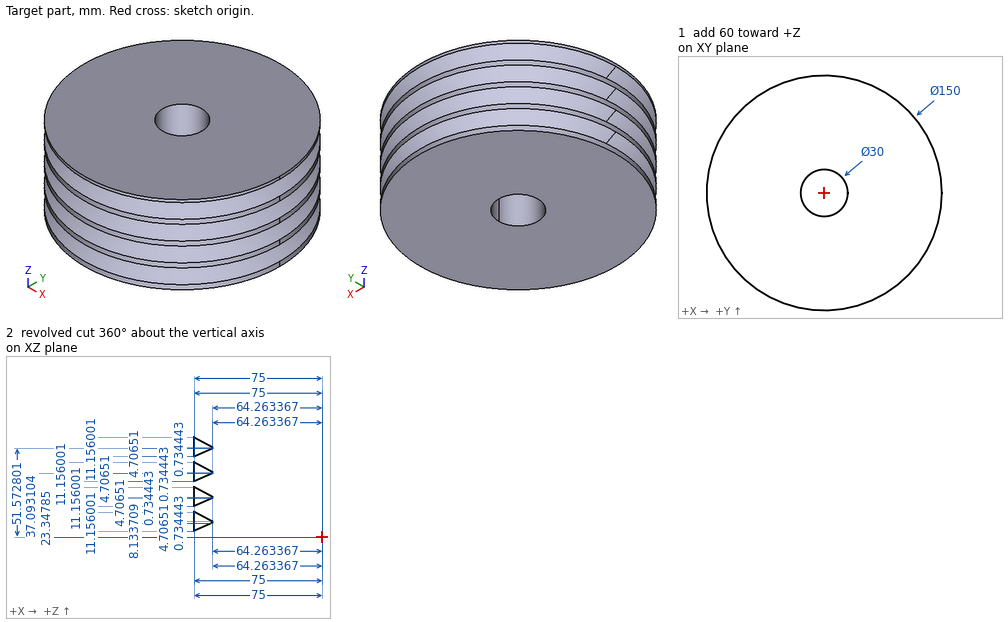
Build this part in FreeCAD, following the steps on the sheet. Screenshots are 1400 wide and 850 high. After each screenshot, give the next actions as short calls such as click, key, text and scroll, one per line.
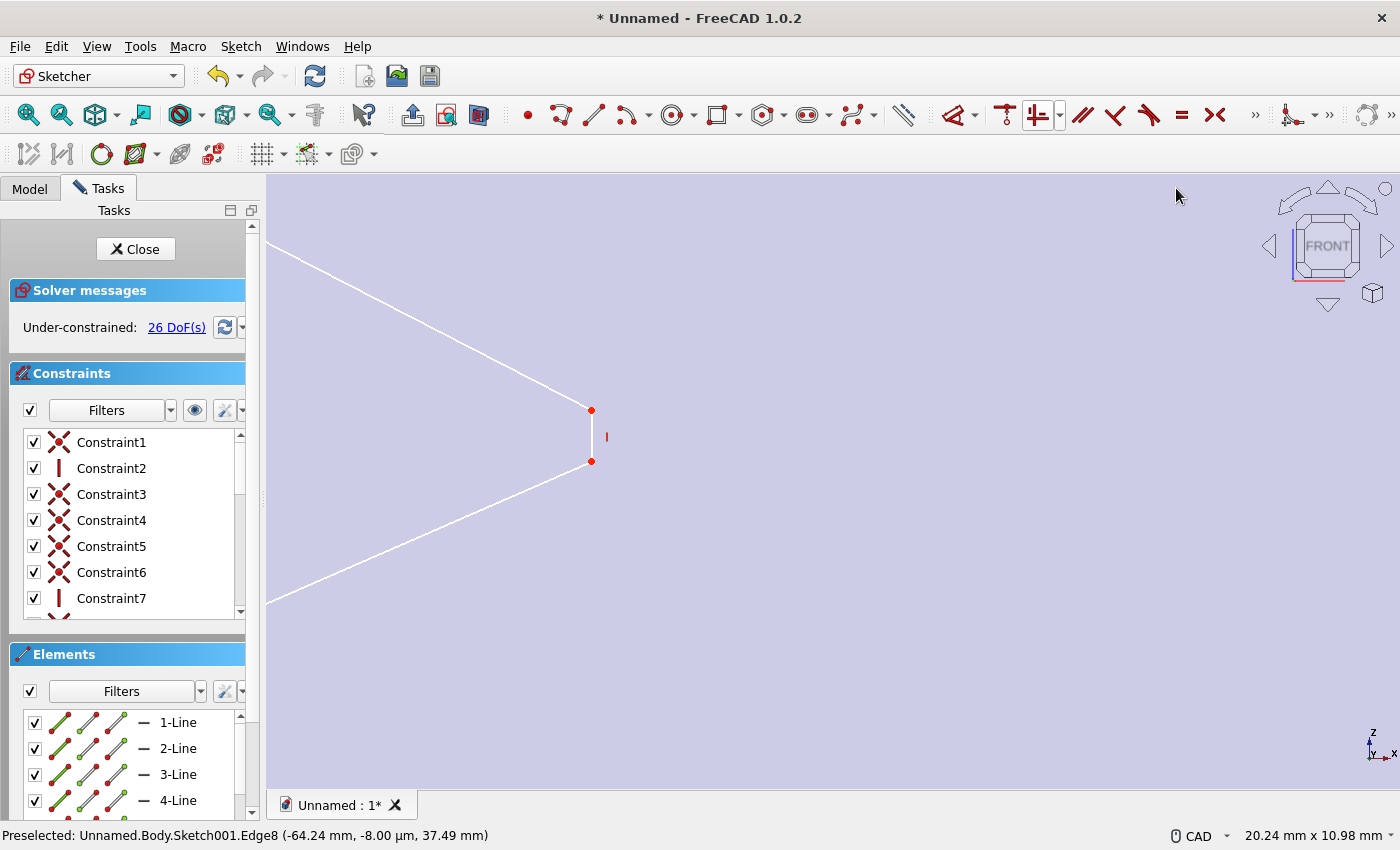
scroll(599, 429, down, 11)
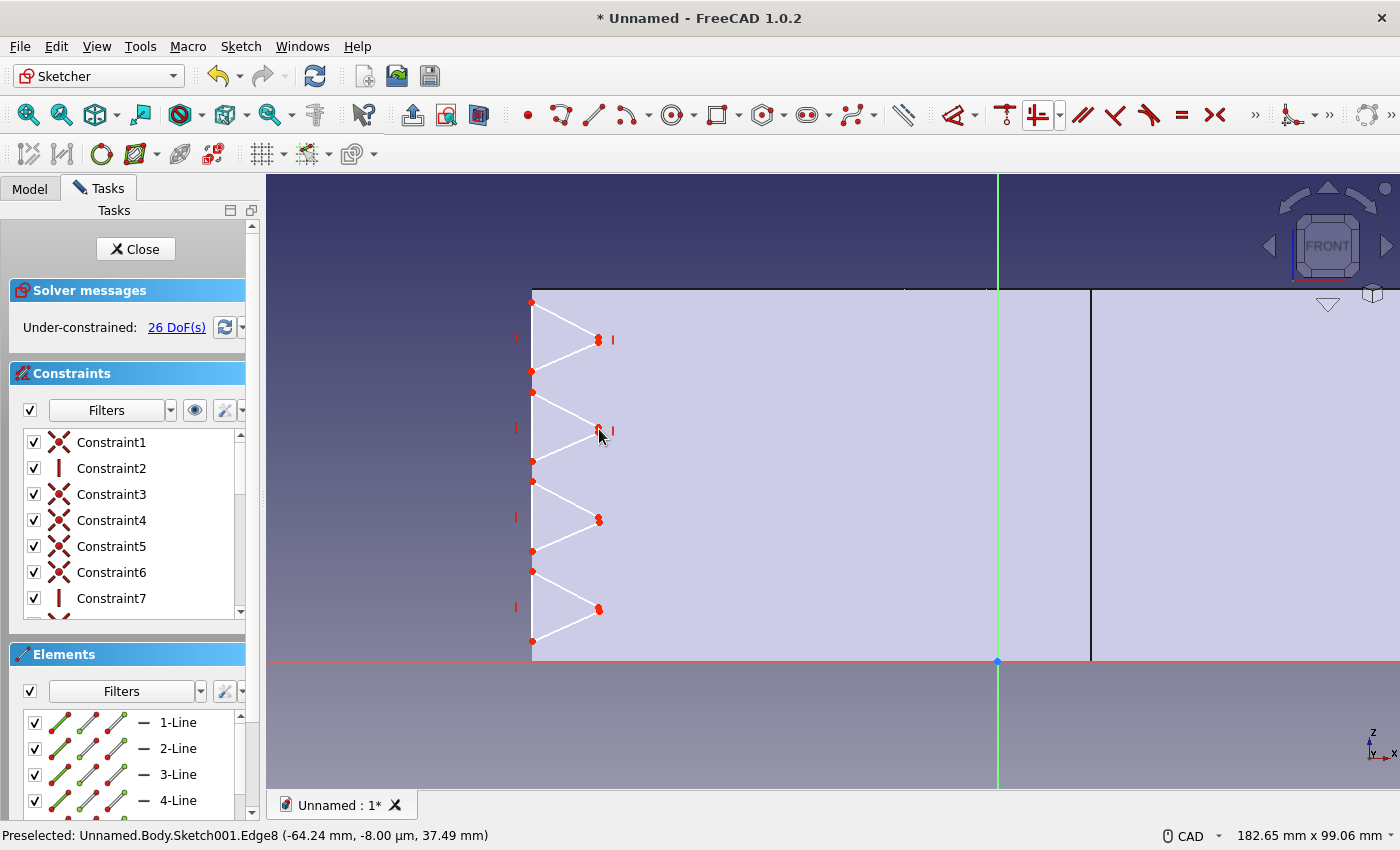
scroll(599, 519, up, 11)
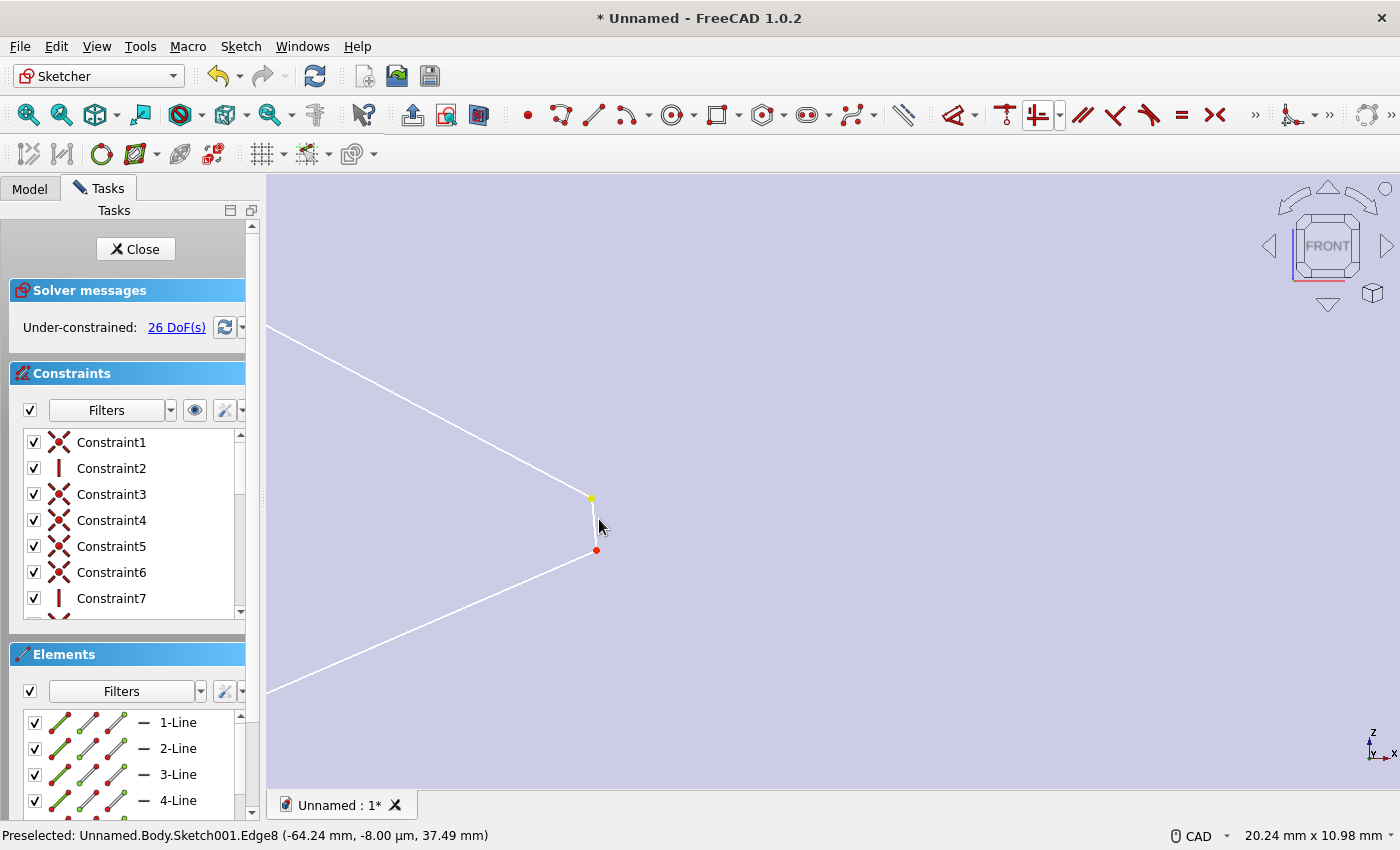
click(593, 514)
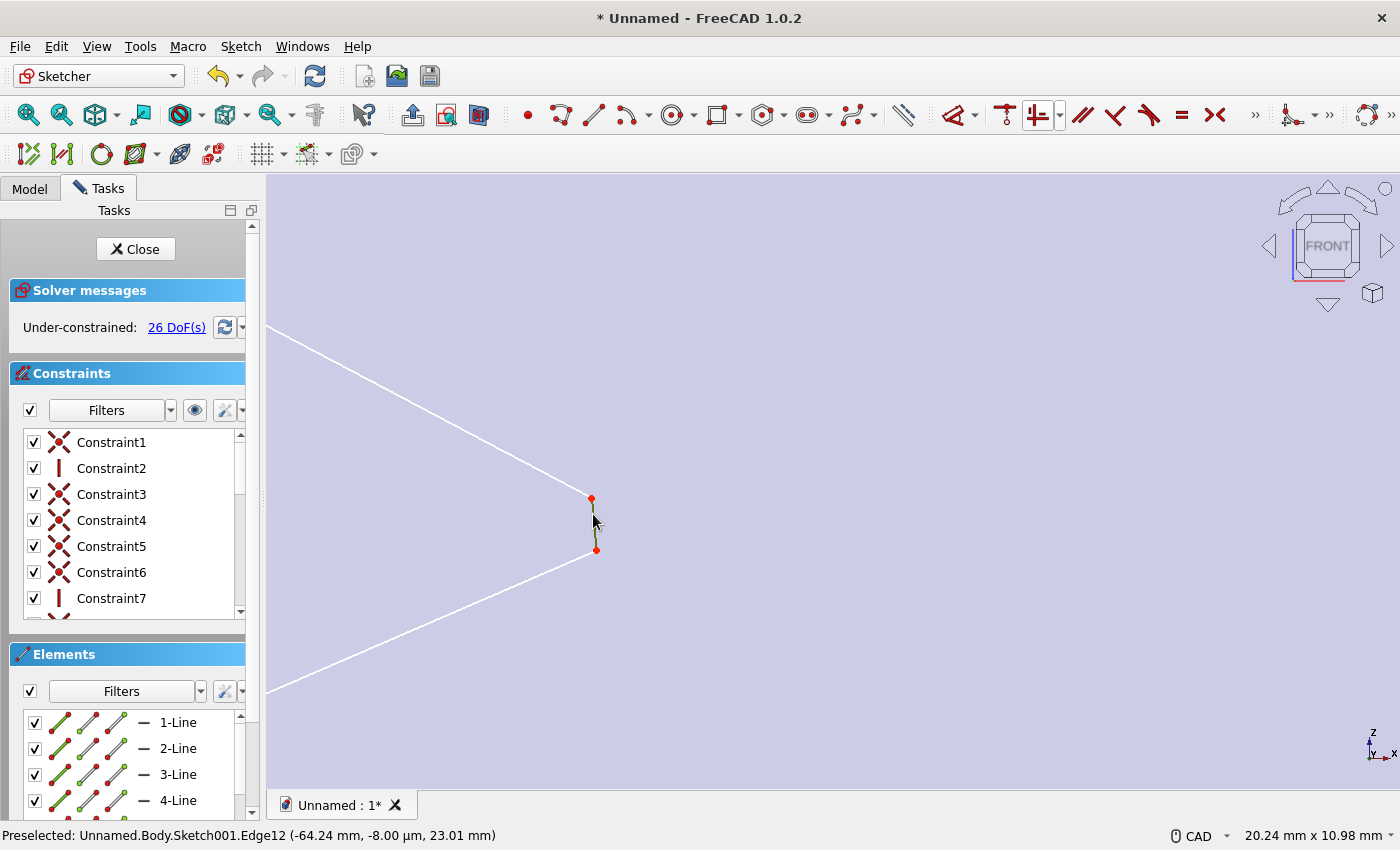
click(1060, 116)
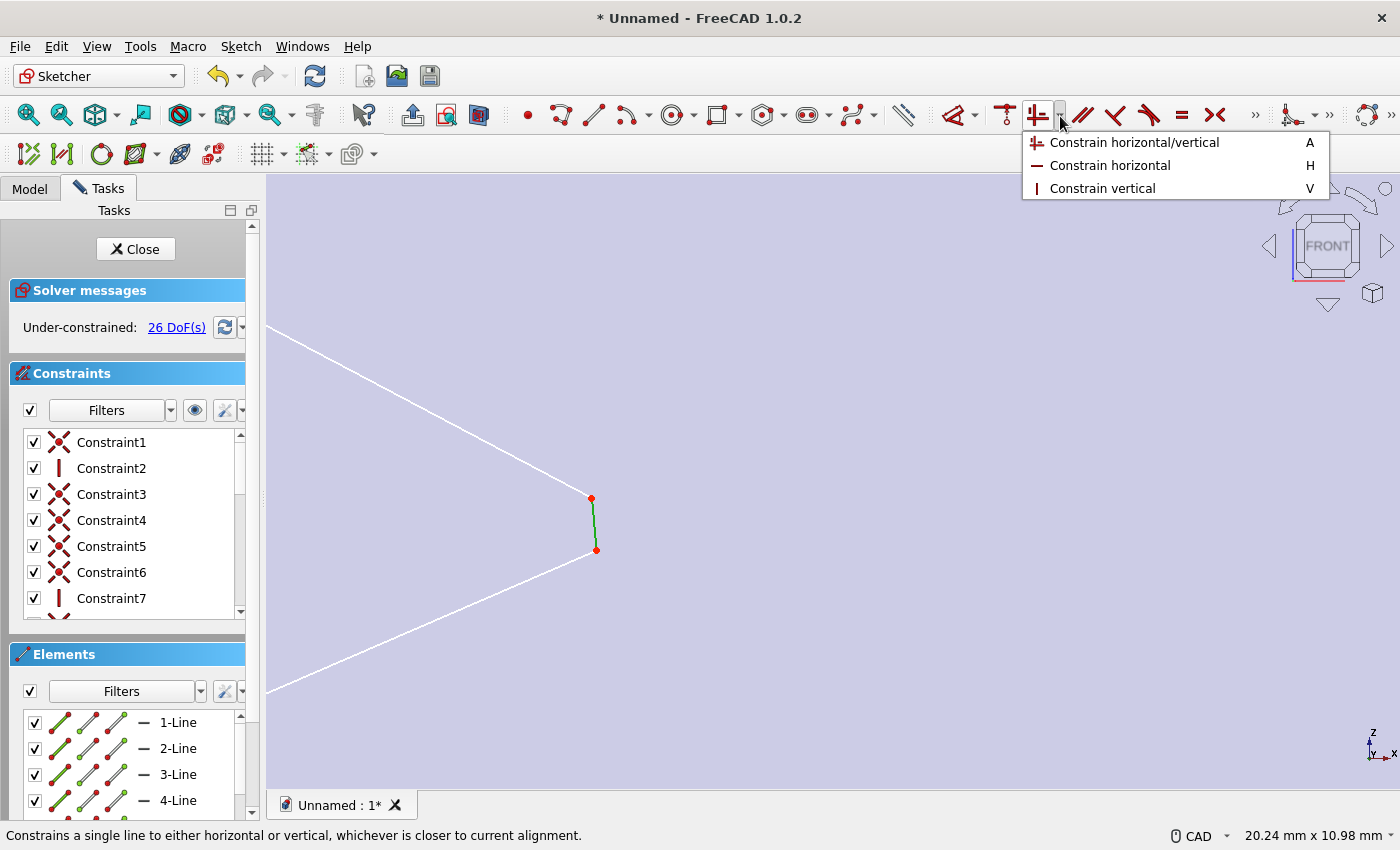
click(1176, 188)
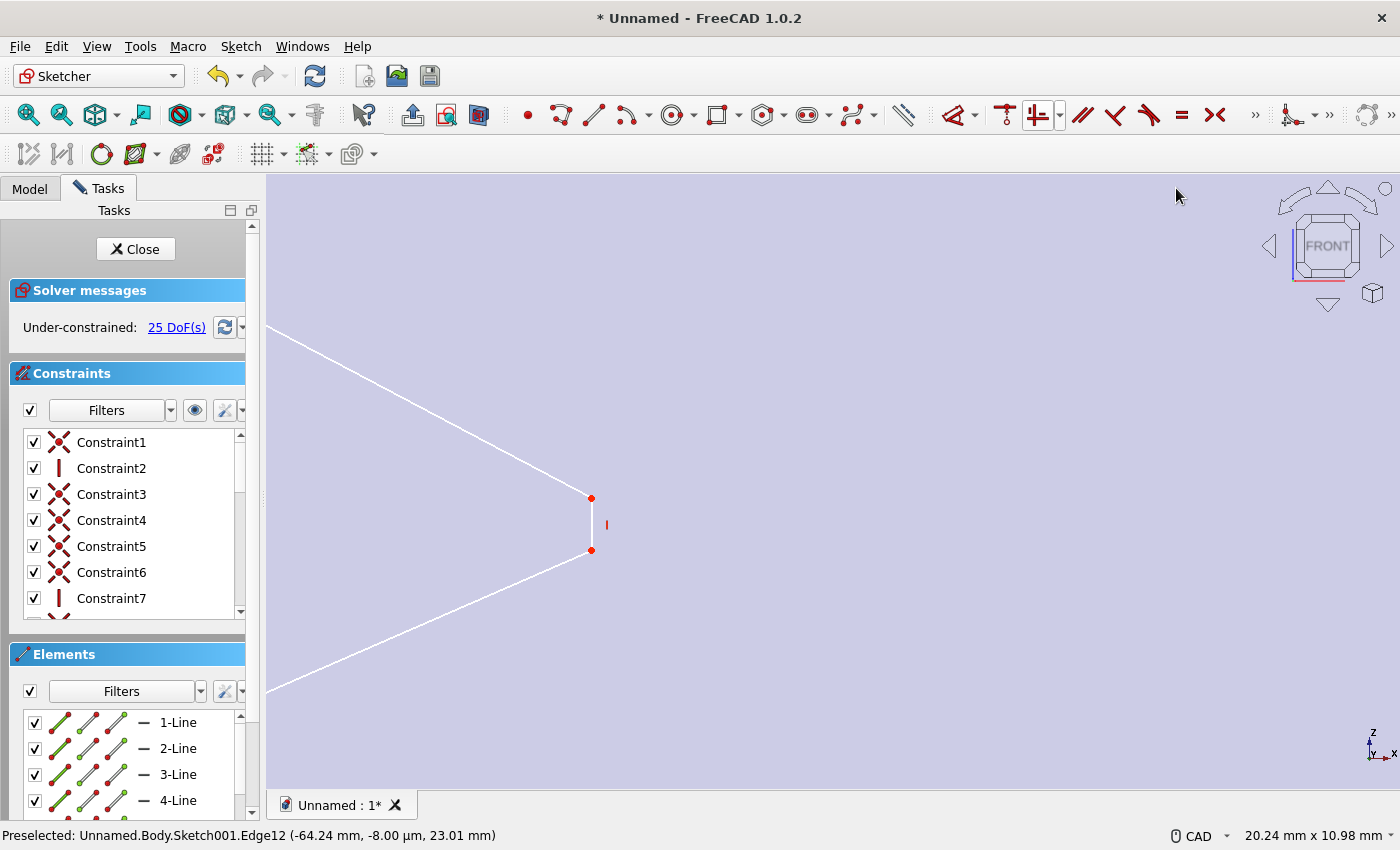
scroll(599, 519, down, 11)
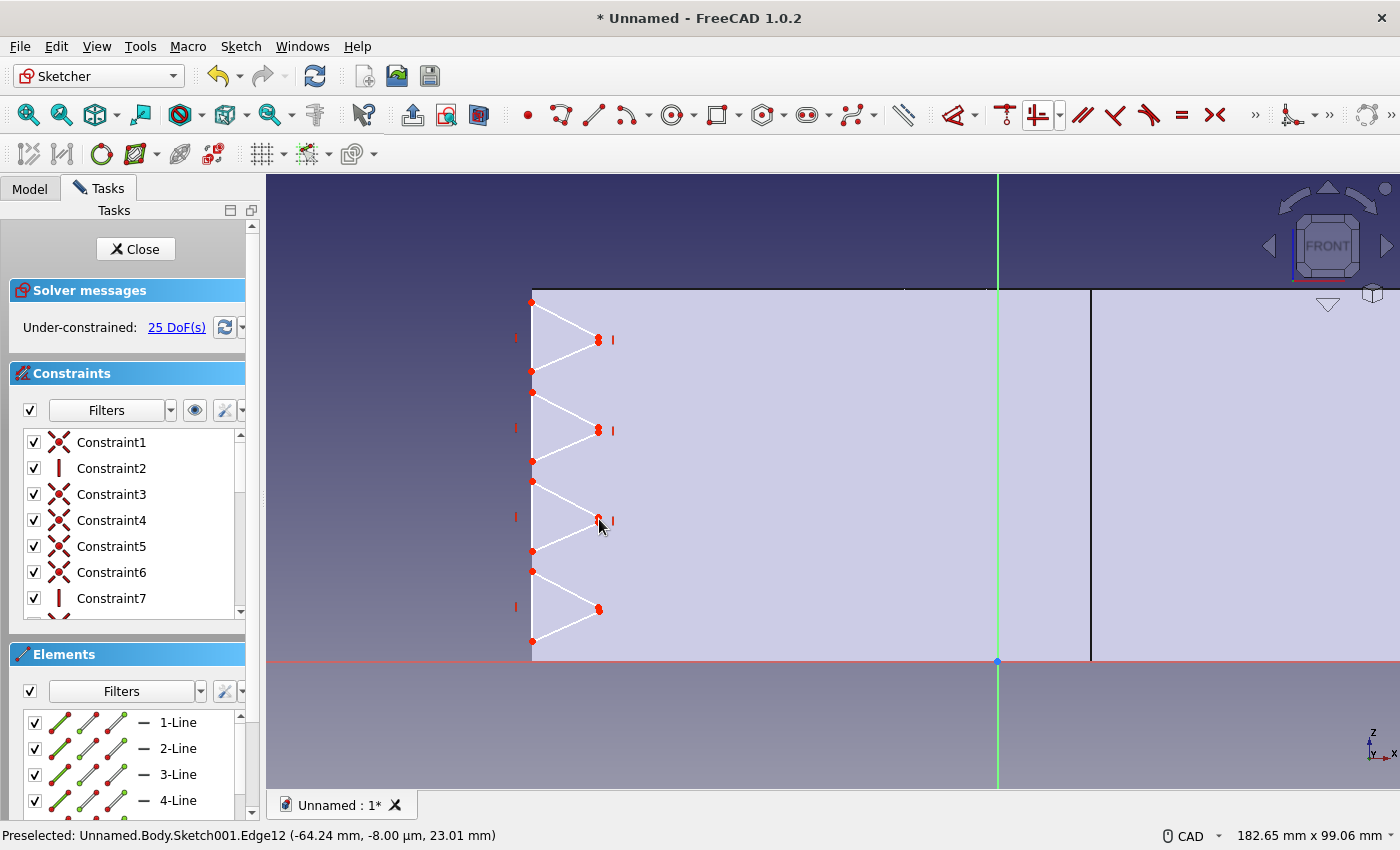
scroll(599, 609, up, 12)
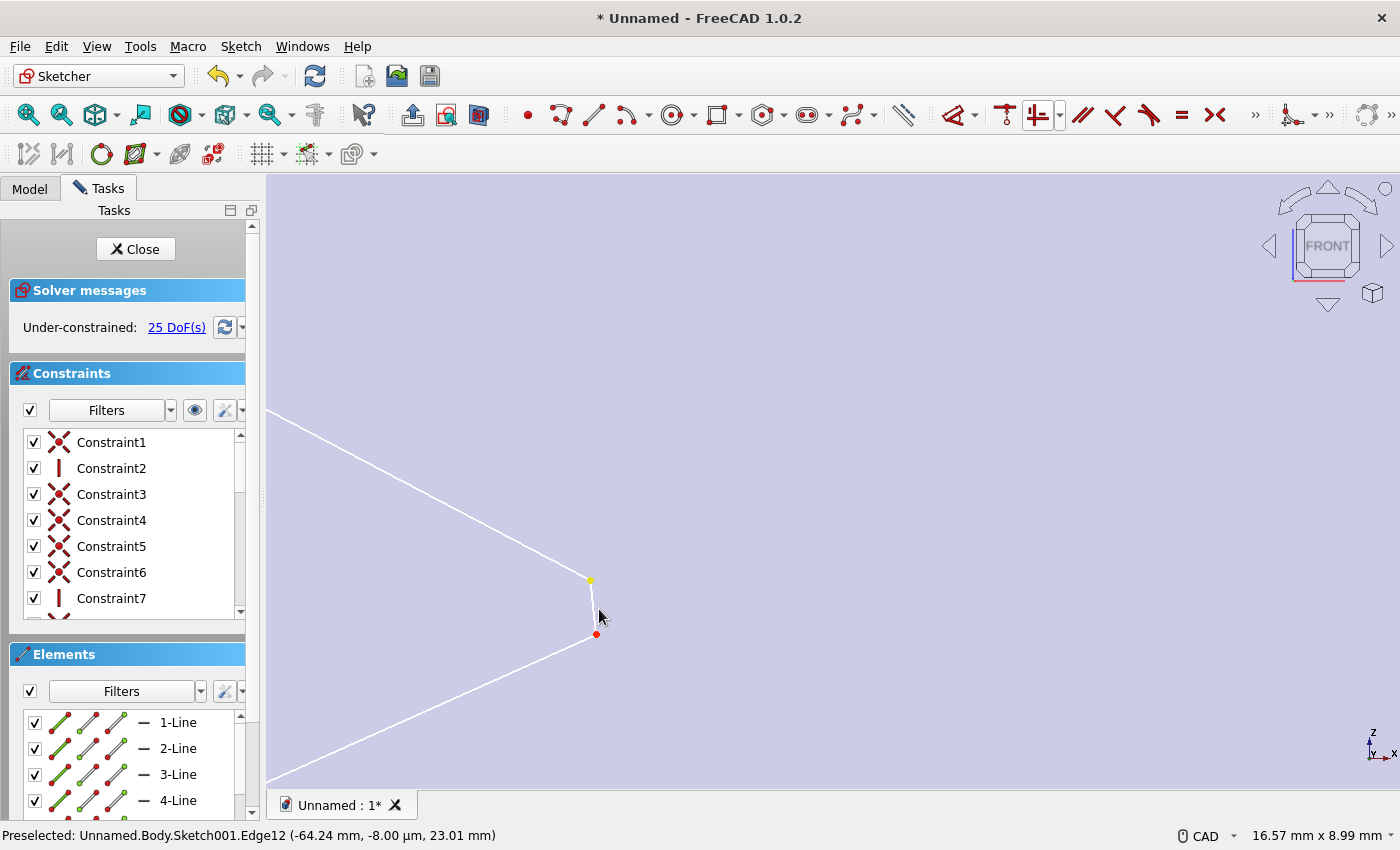
click(592, 597)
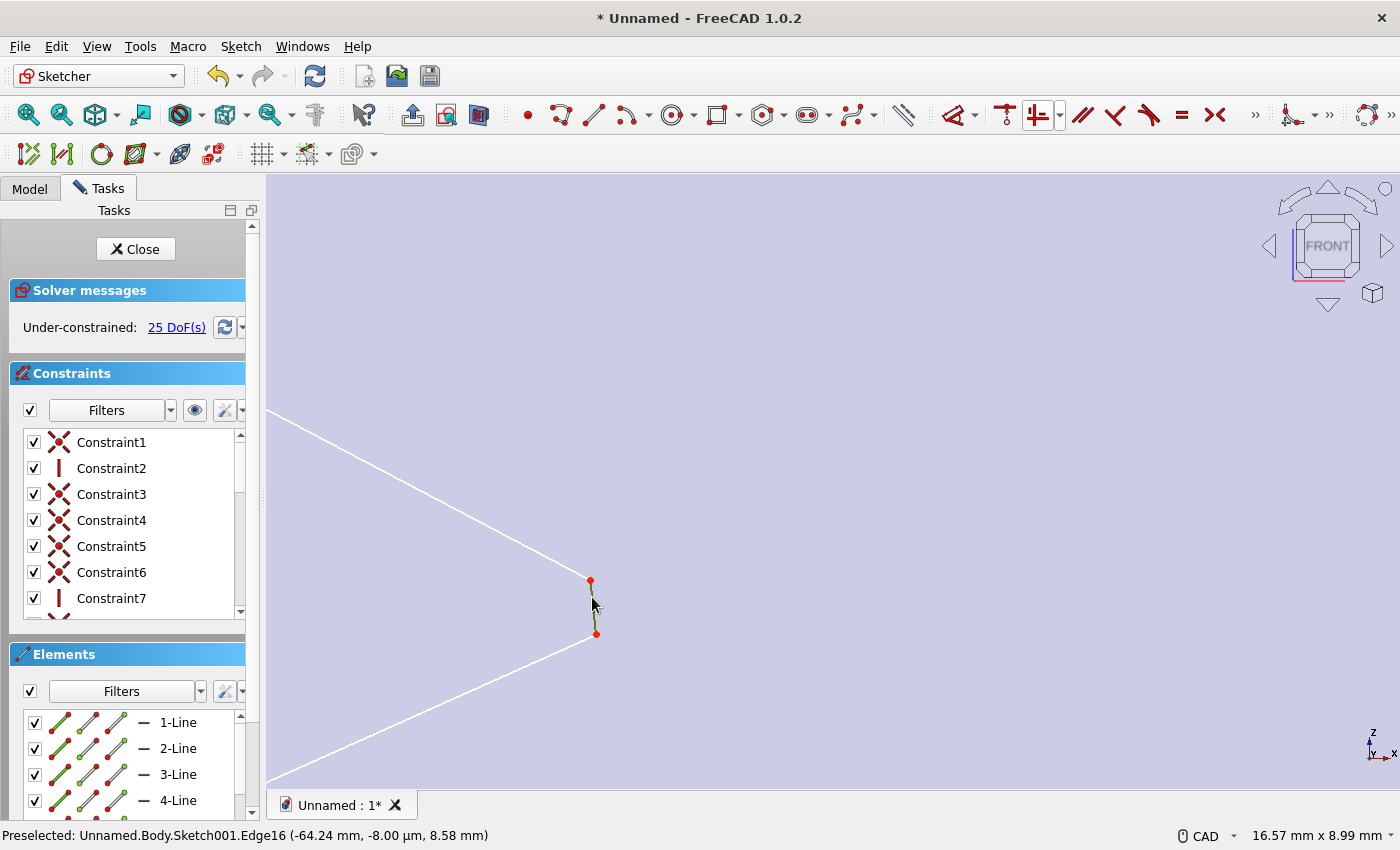
click(1060, 116)